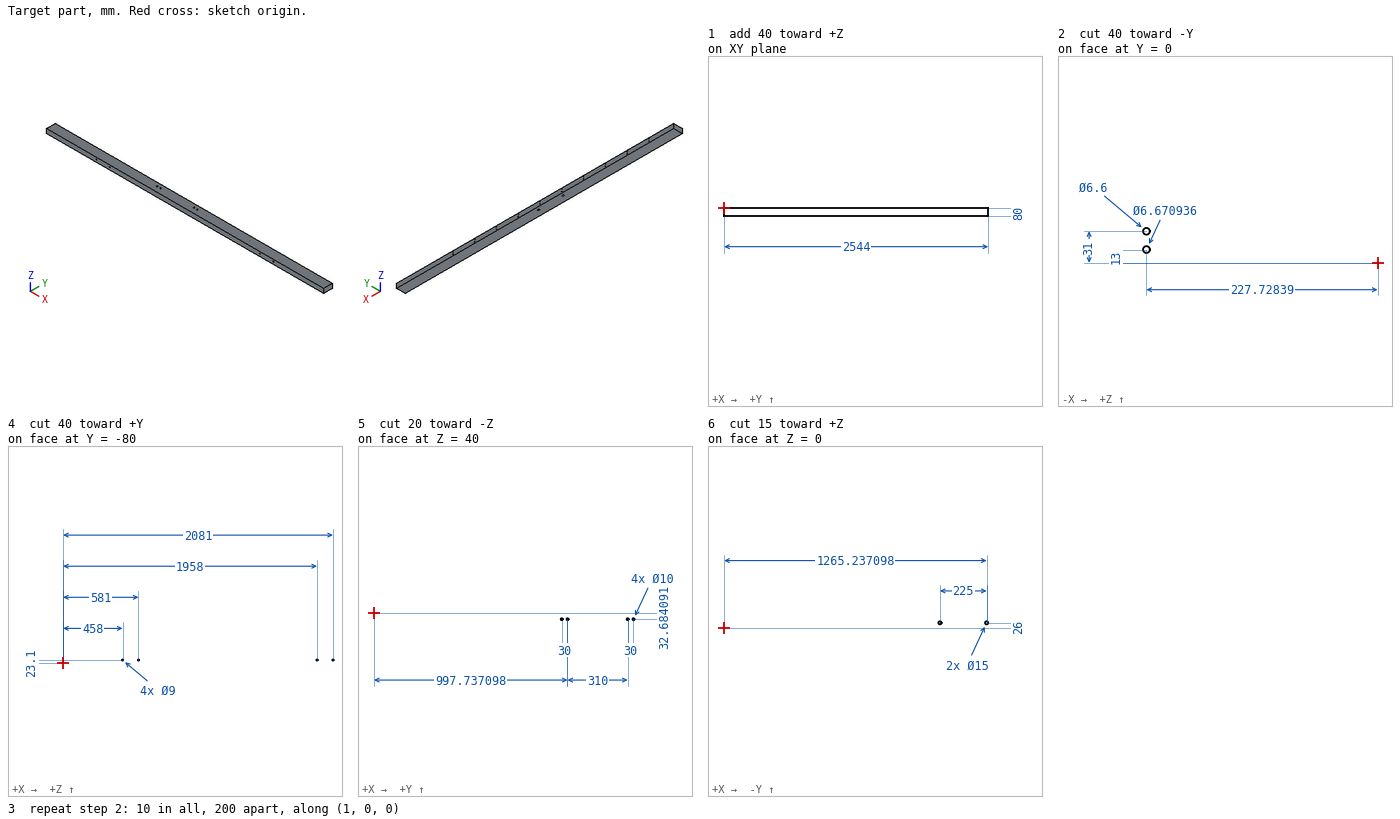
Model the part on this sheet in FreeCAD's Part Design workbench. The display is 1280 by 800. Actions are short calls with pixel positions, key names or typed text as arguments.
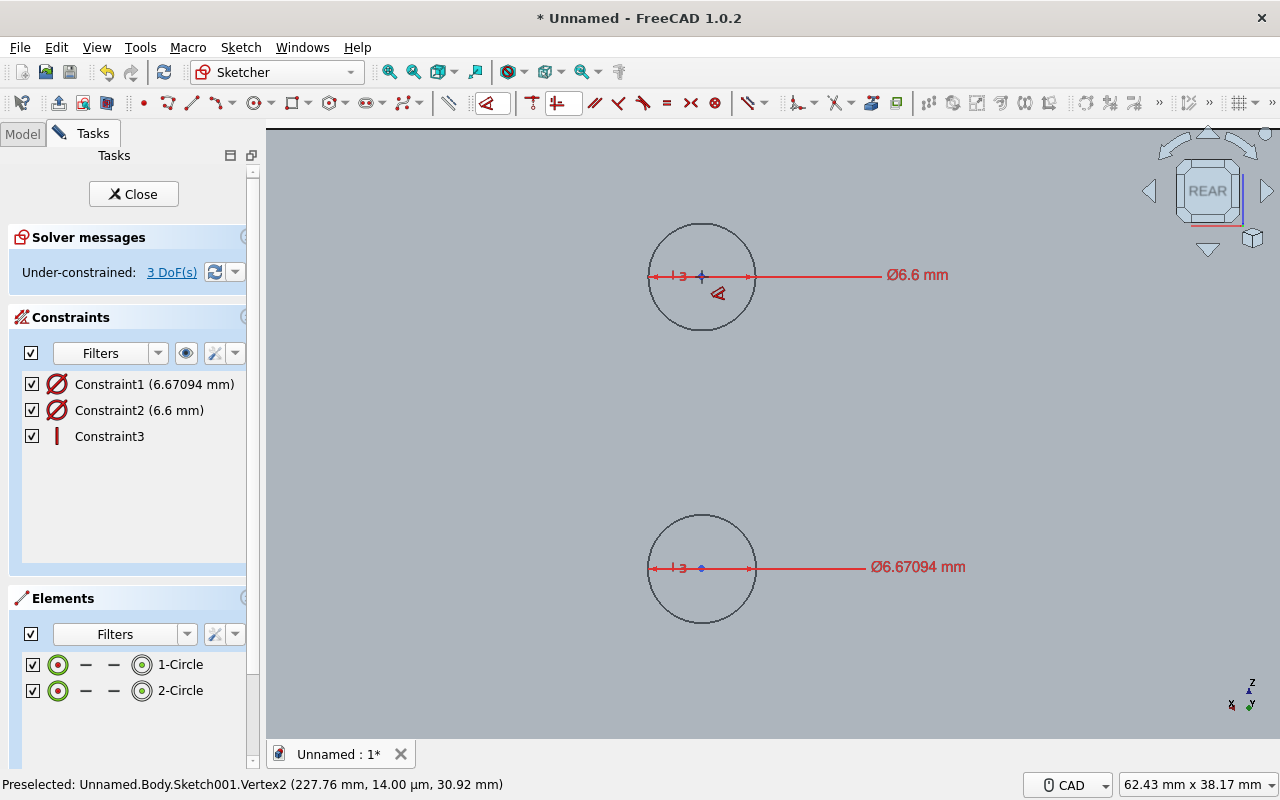
click(702, 569)
click(668, 640)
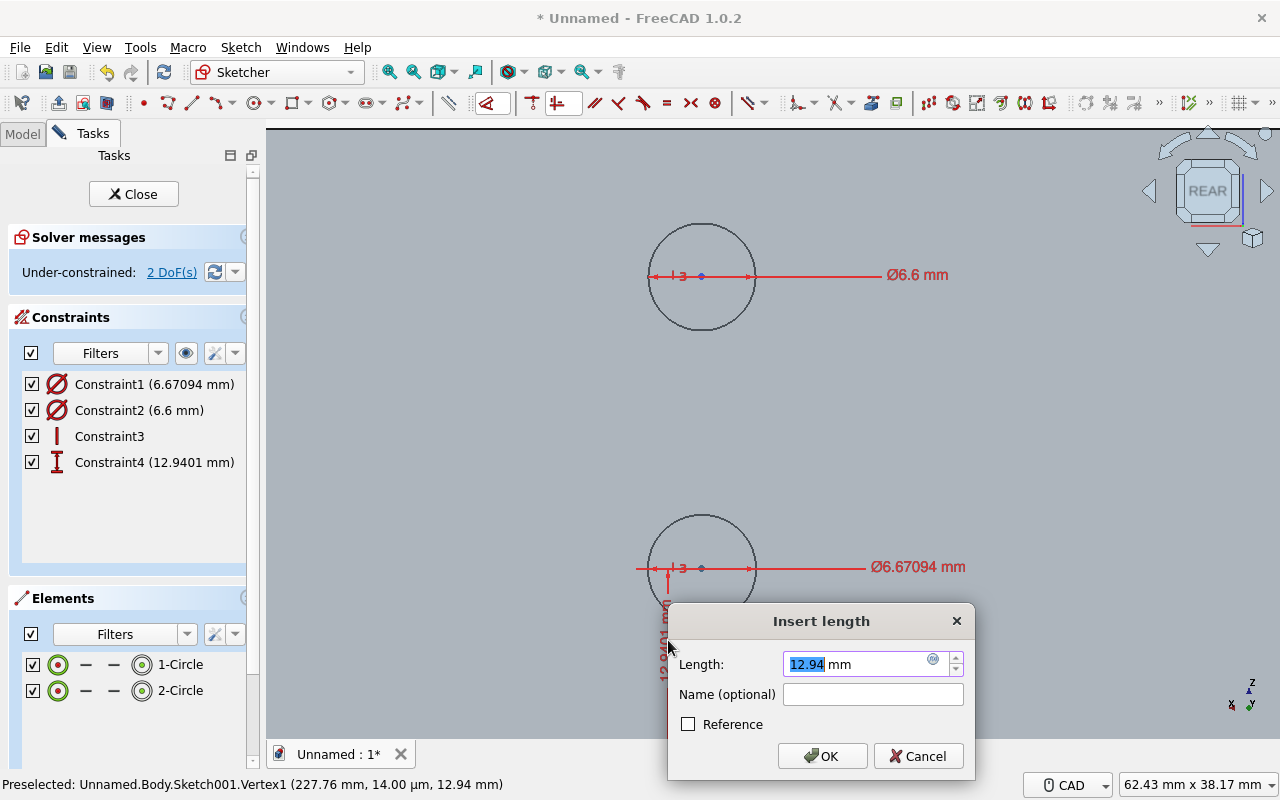
text(13)
key(Return)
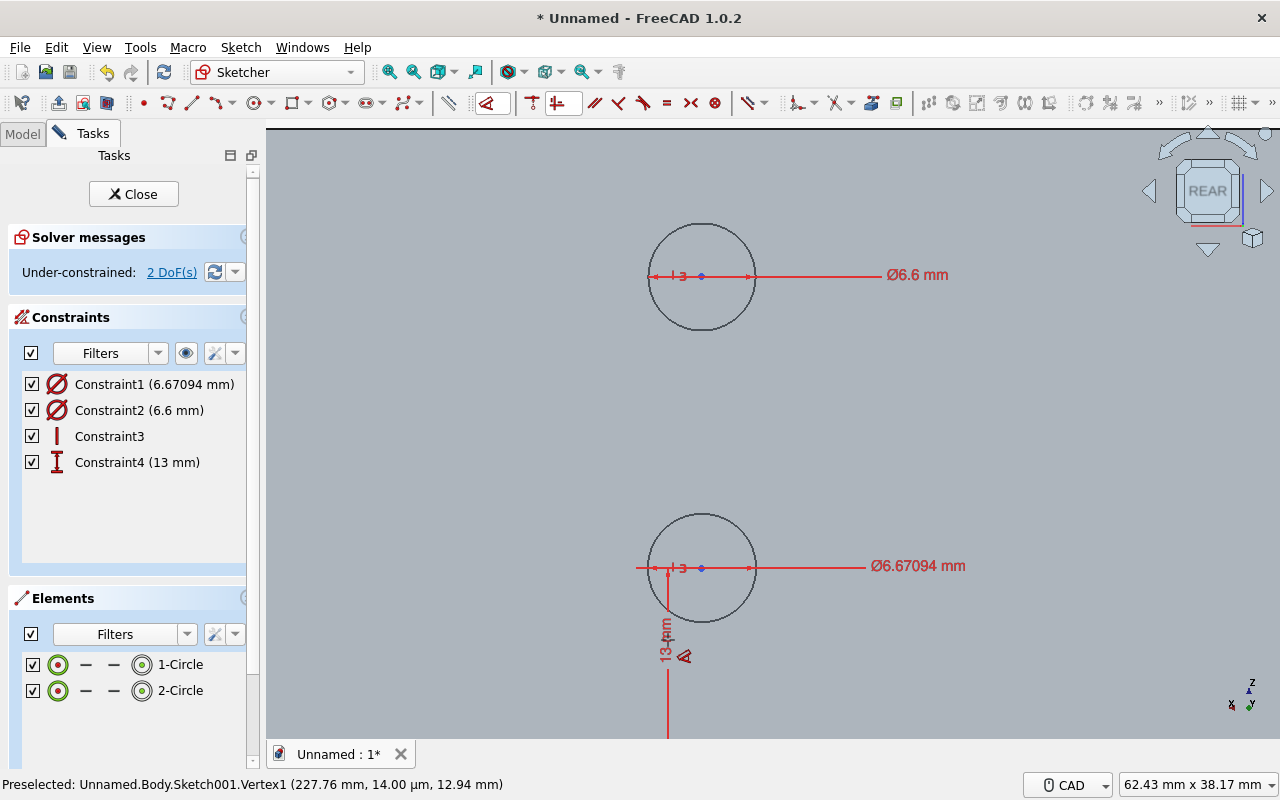
click(702, 277)
click(668, 494)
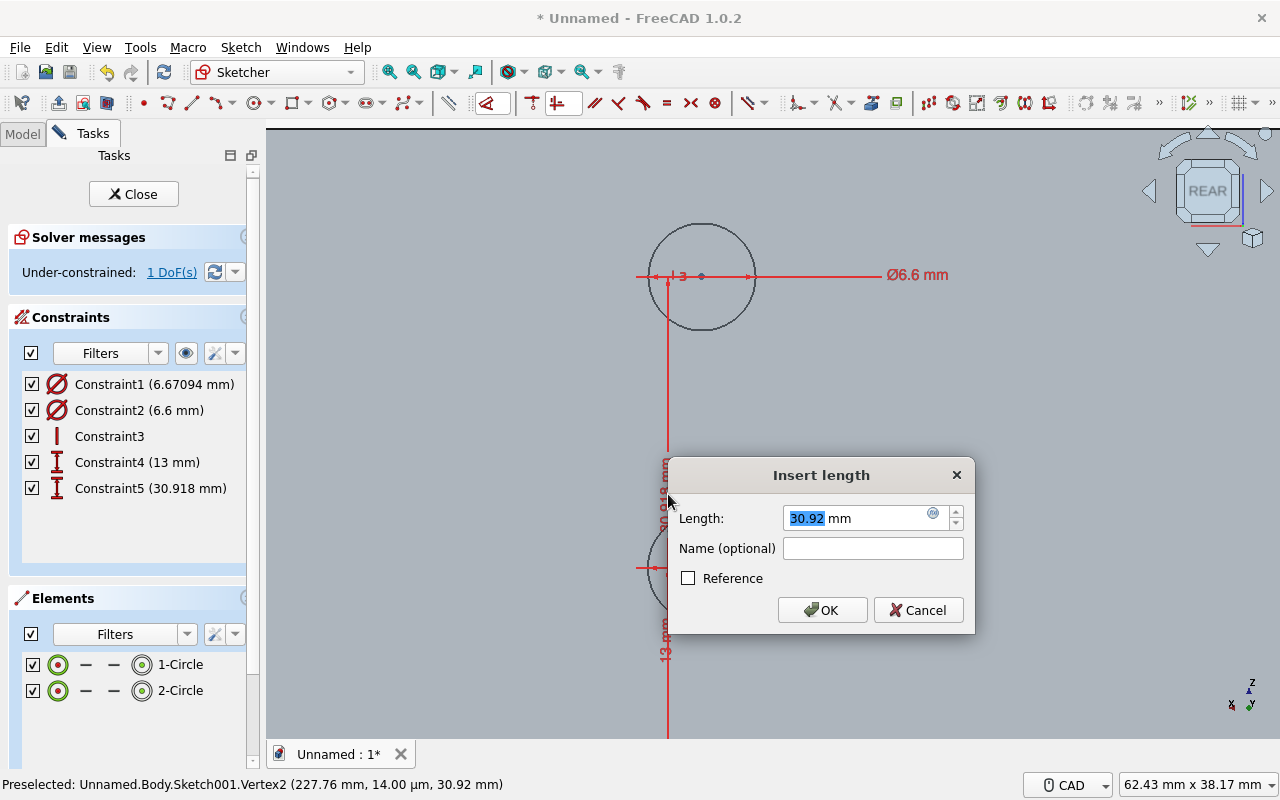
text(31)
key(Return)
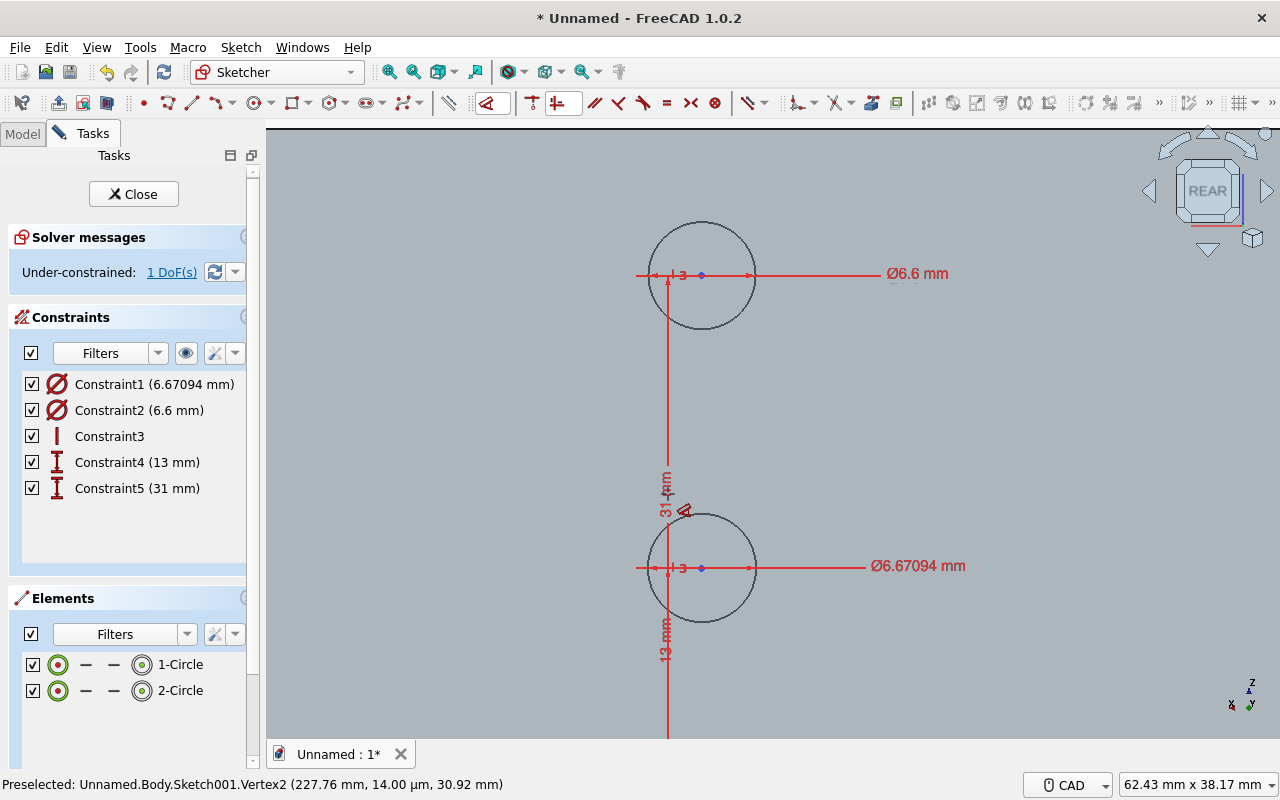
click(702, 568)
click(908, 534)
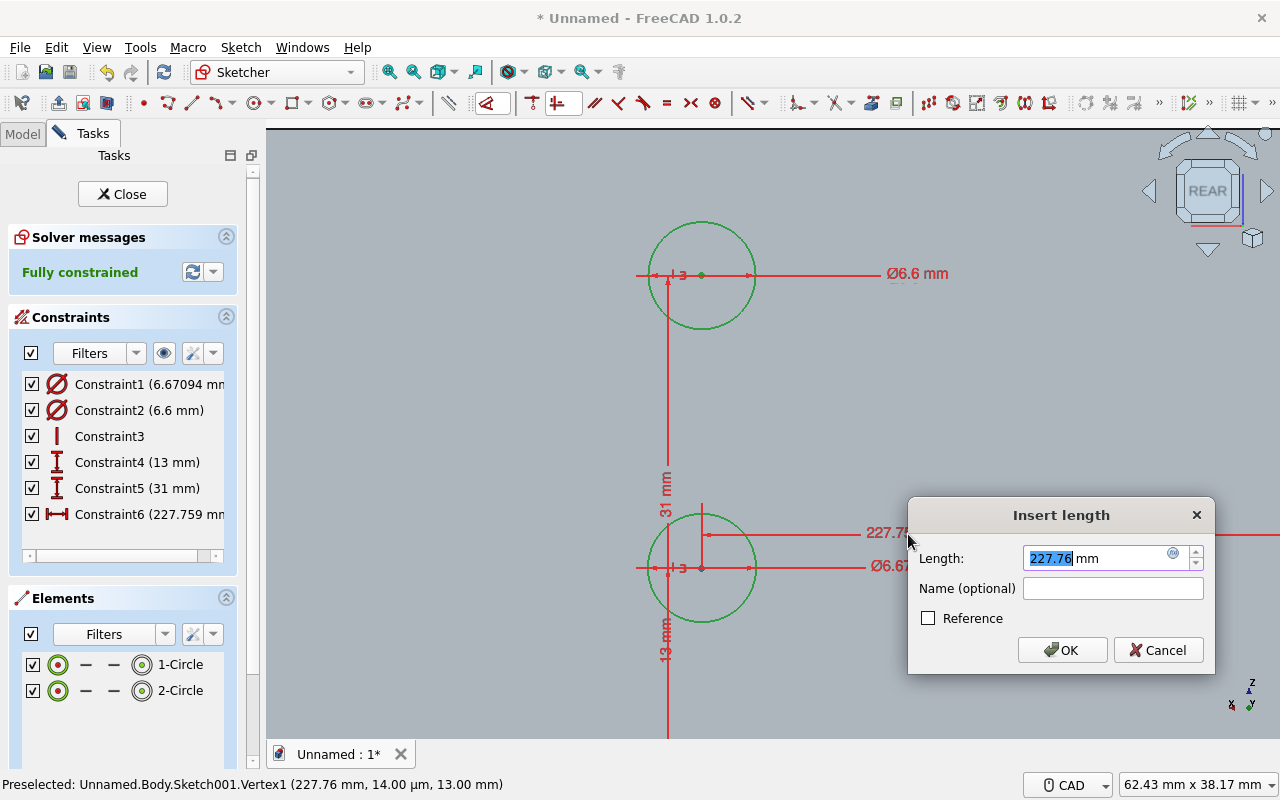
text(227.72839)
key(Return)
key(Escape)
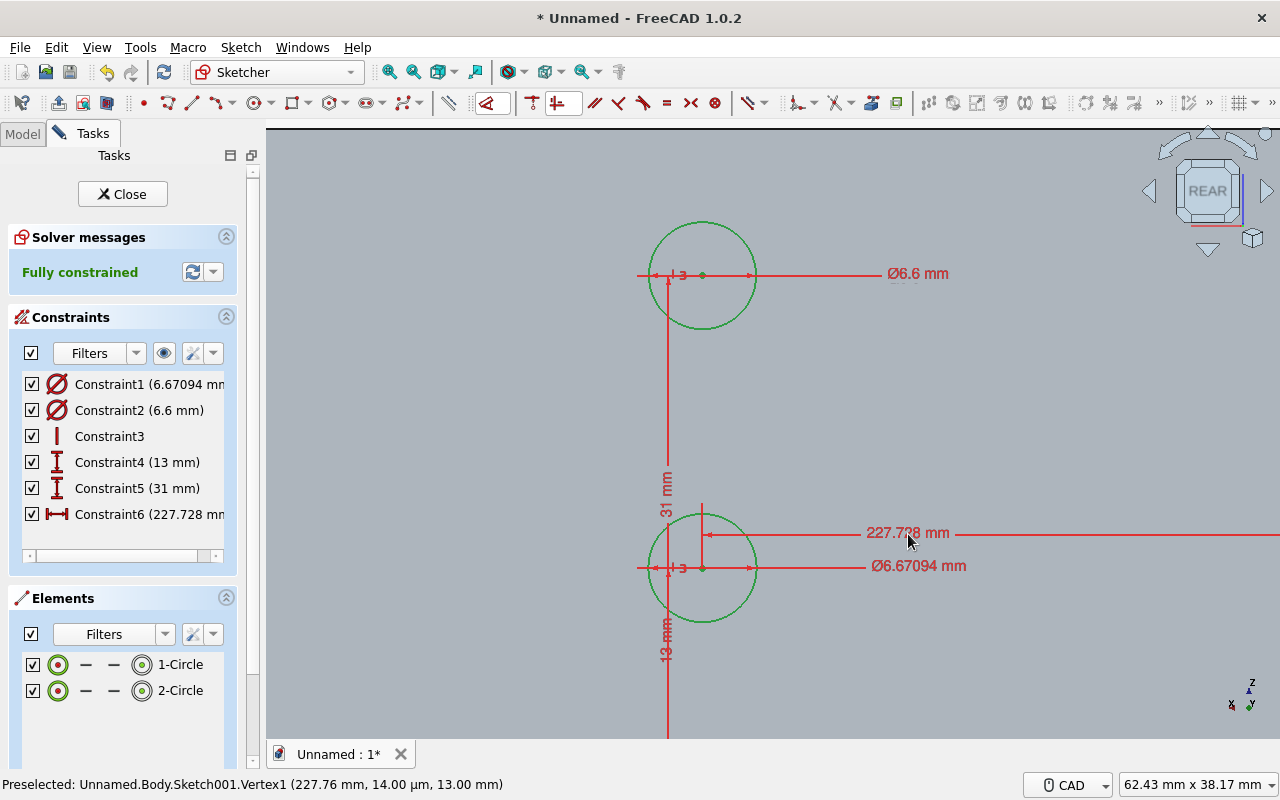
click(123, 194)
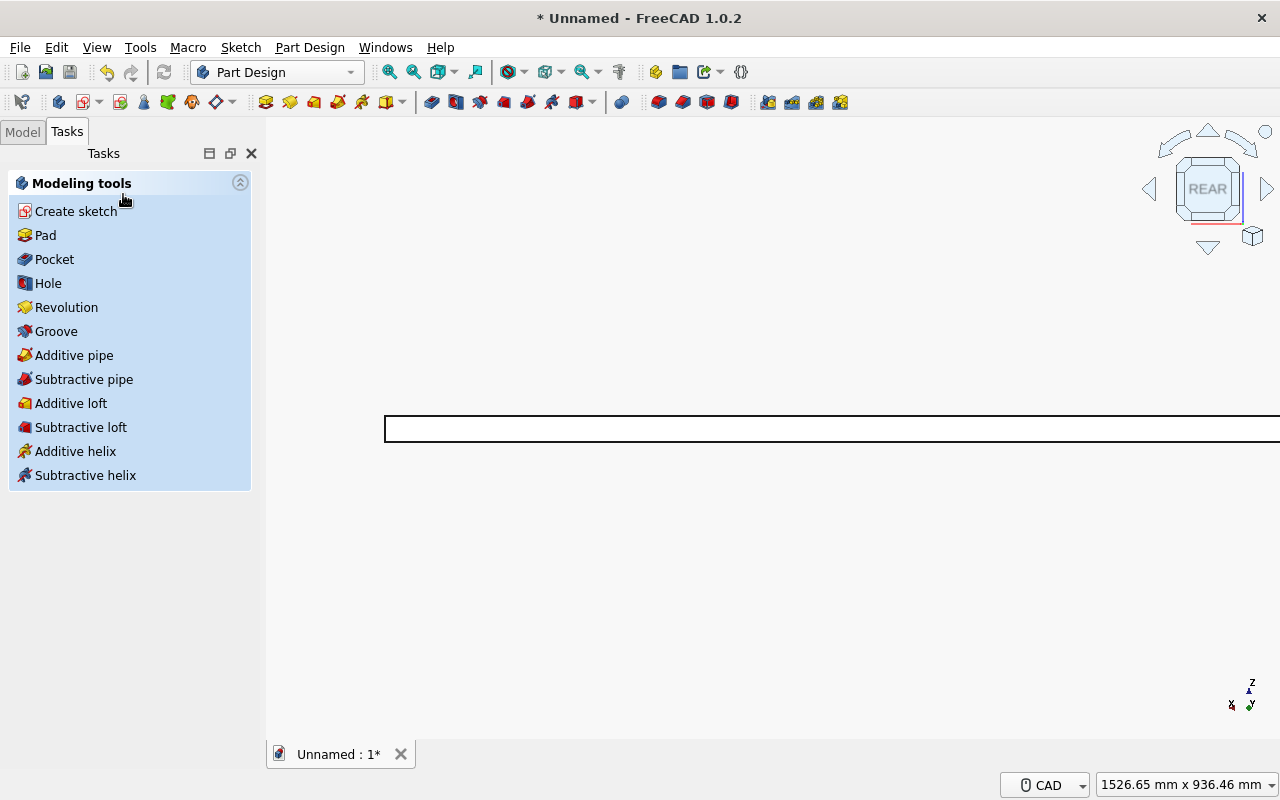
click(432, 102)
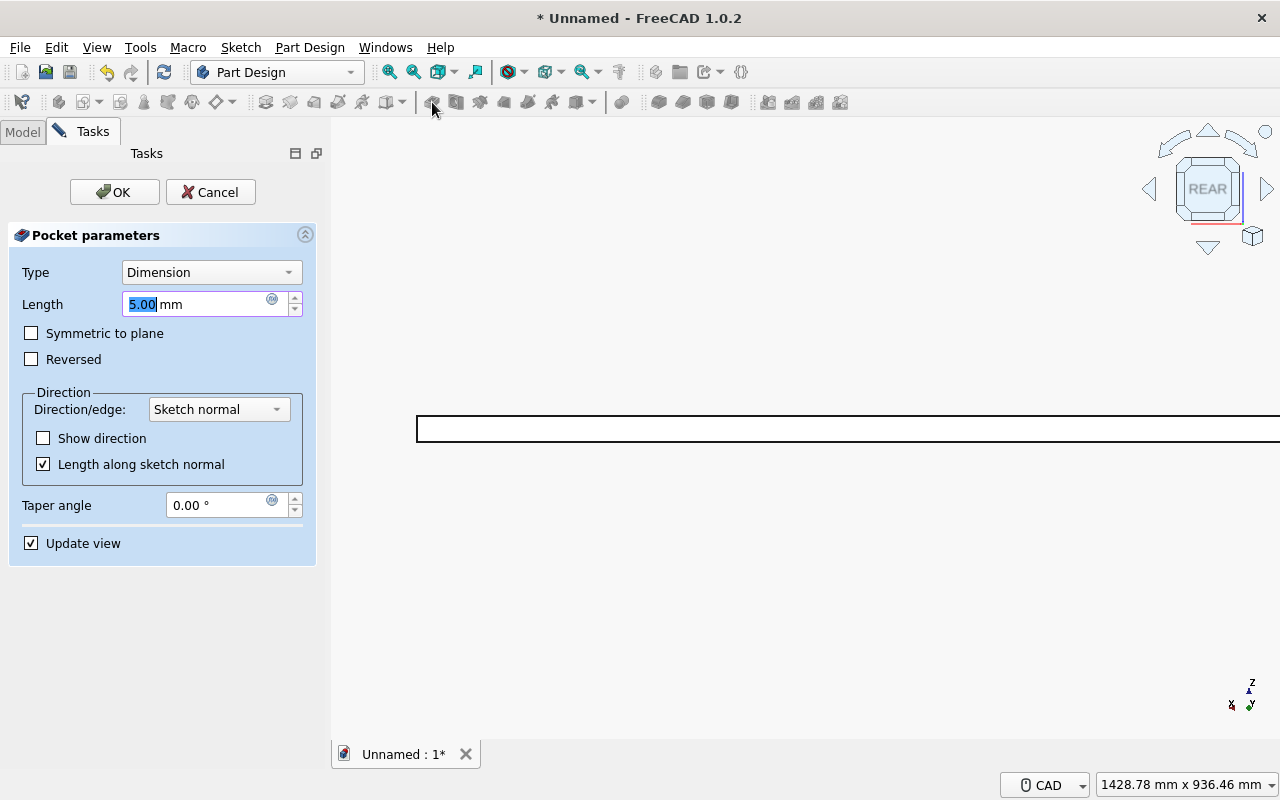
text(40)
key(Tab)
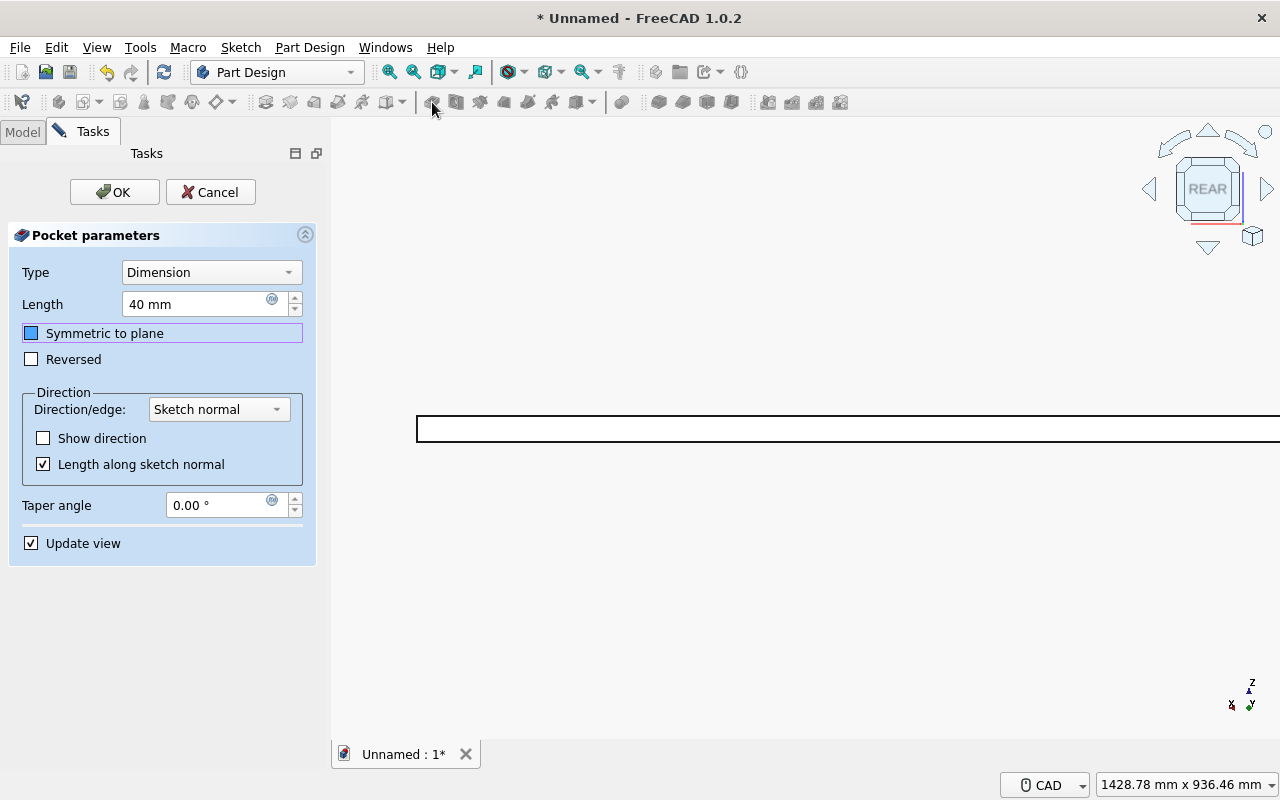
click(115, 192)